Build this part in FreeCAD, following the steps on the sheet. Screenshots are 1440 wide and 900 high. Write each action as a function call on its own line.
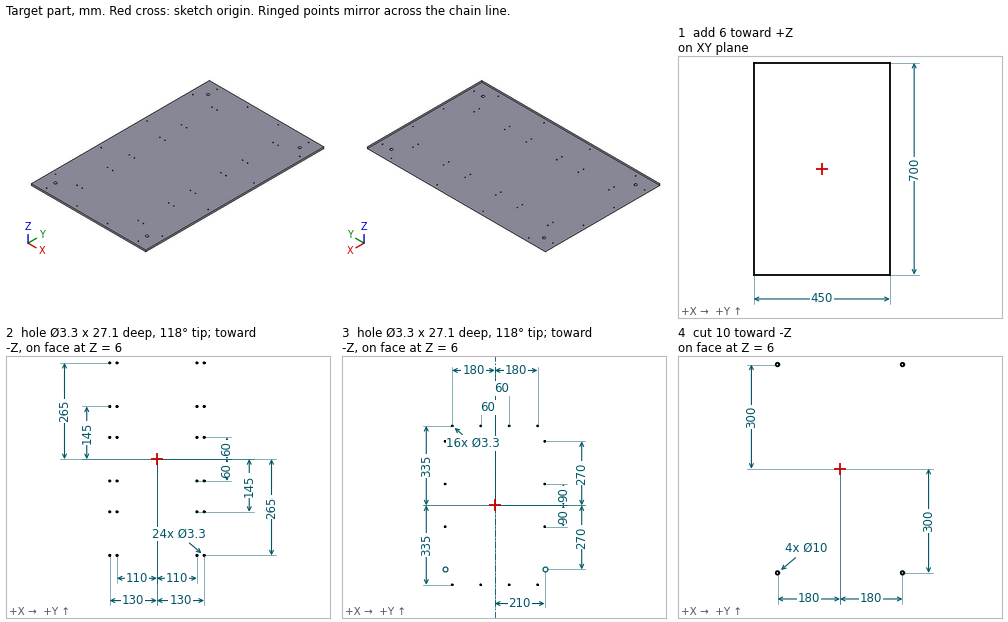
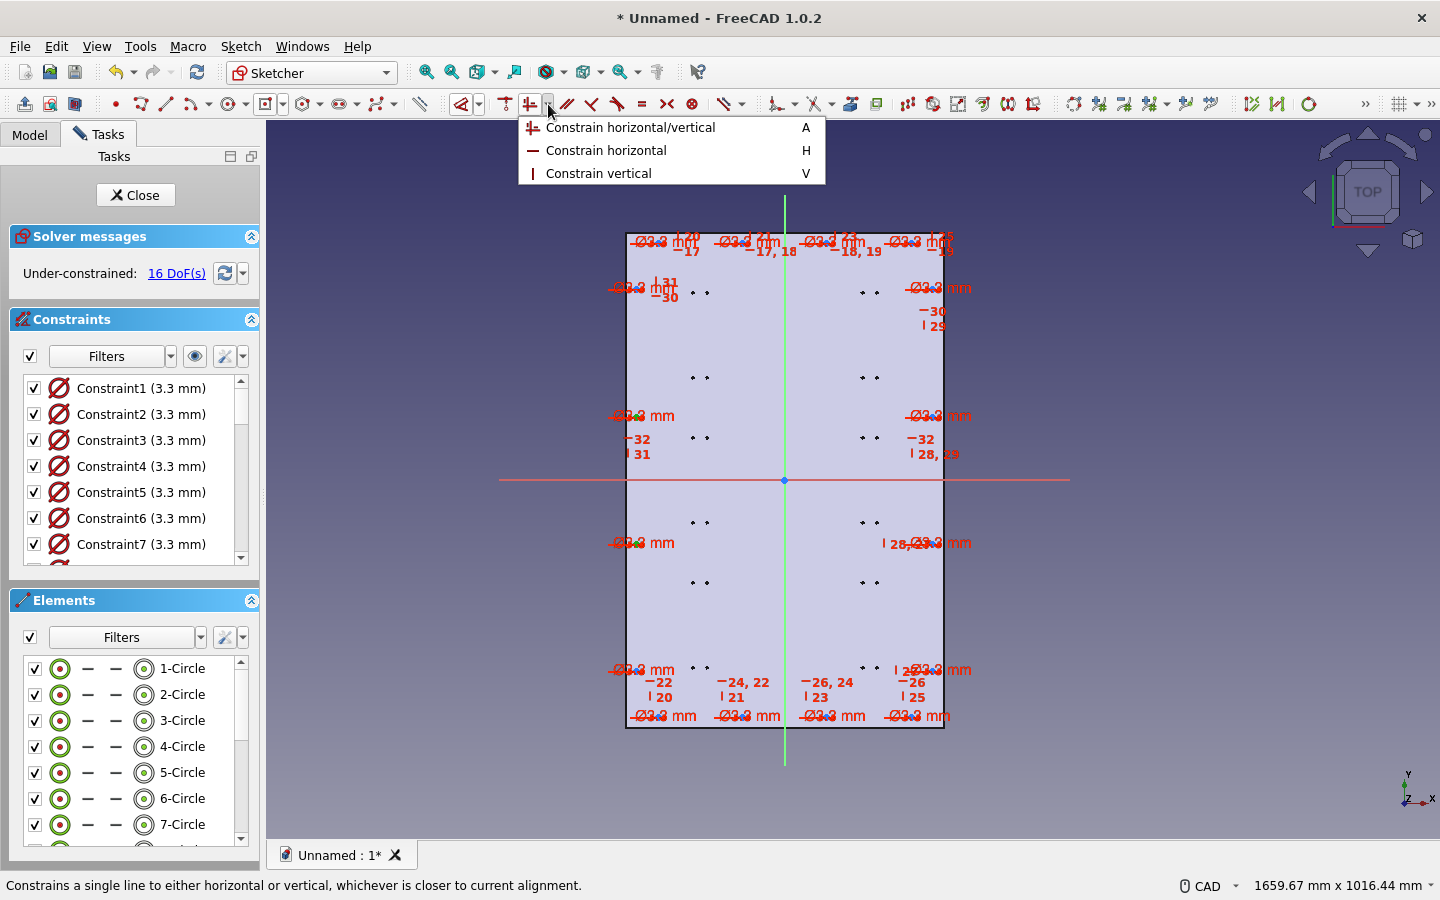
click(672, 174)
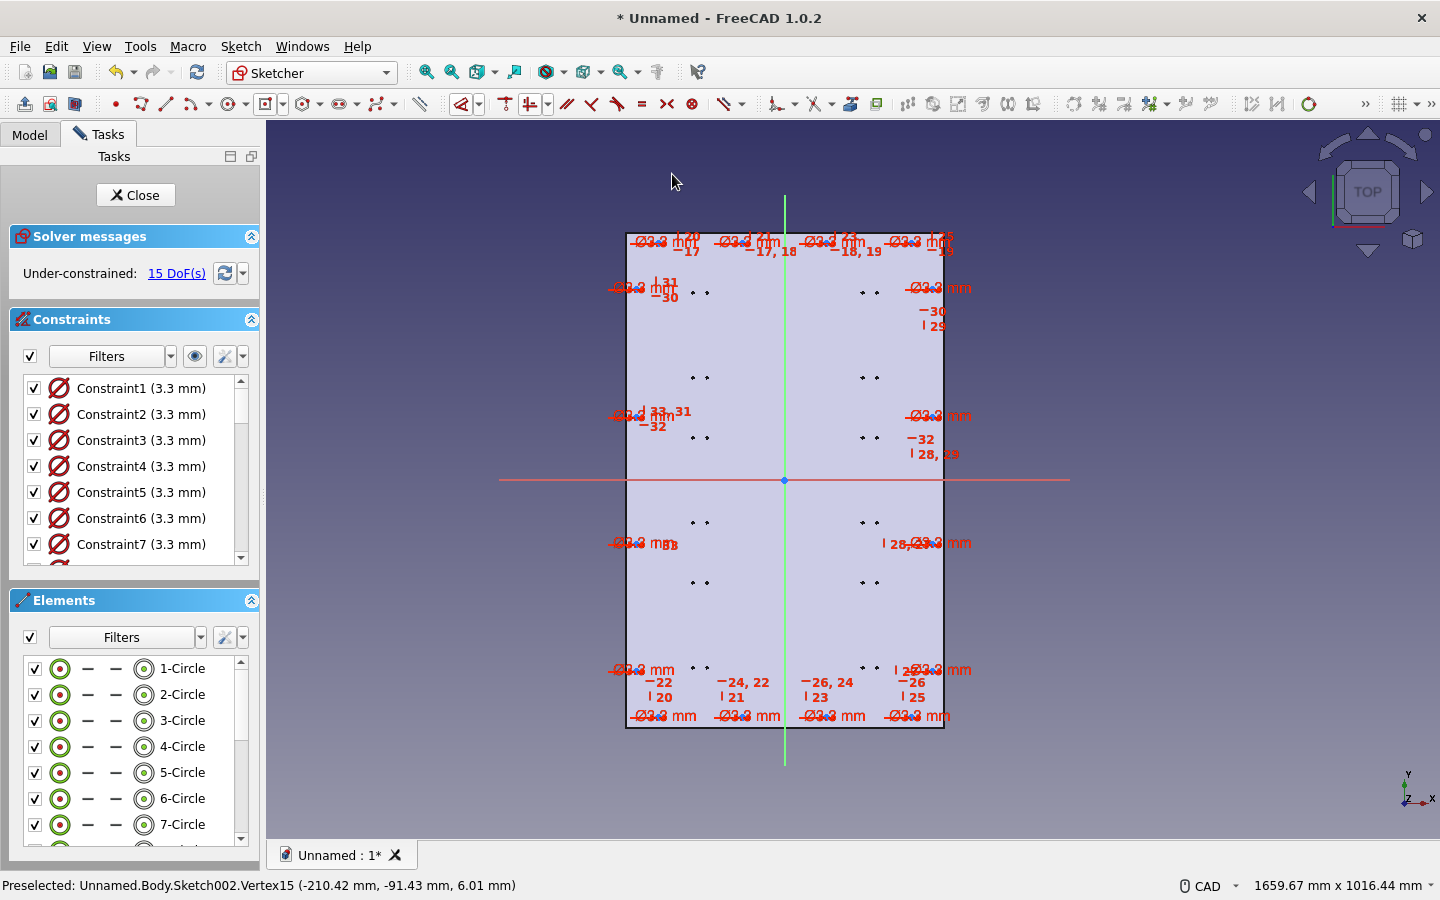
click(933, 545)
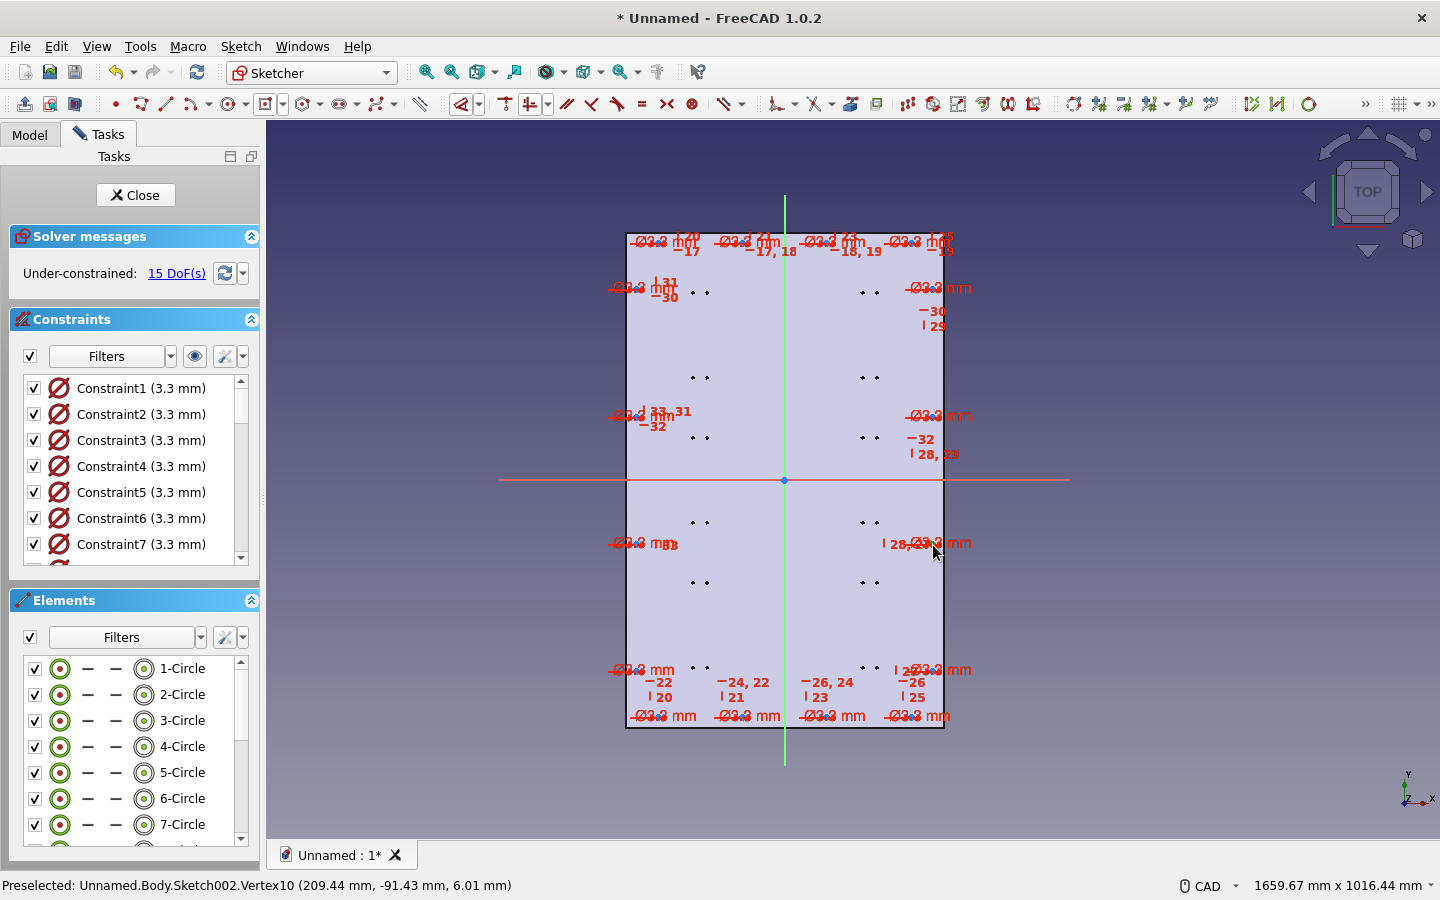
click(636, 545)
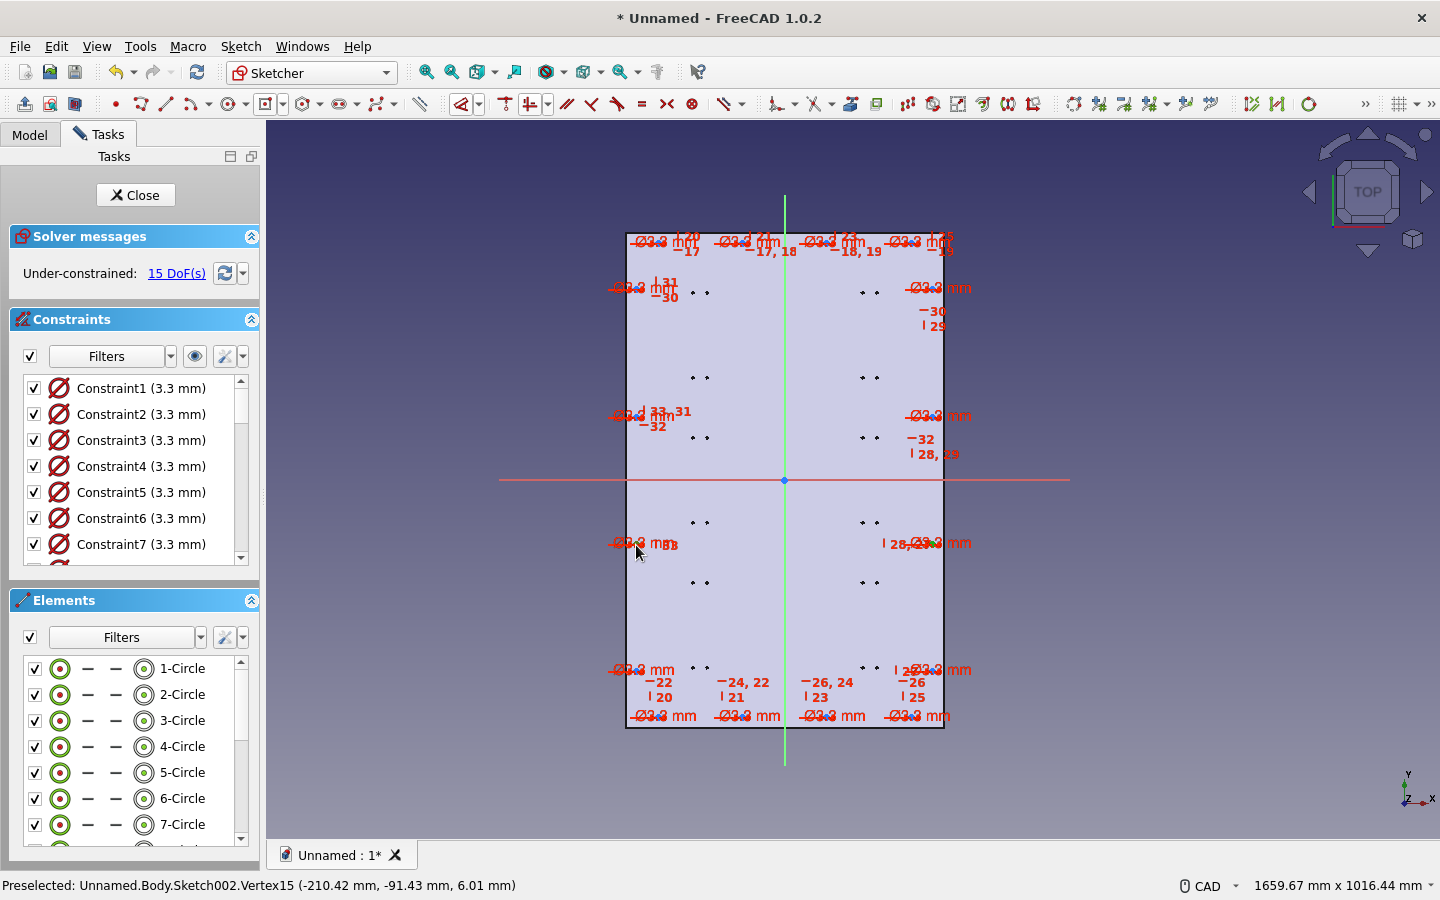
click(548, 104)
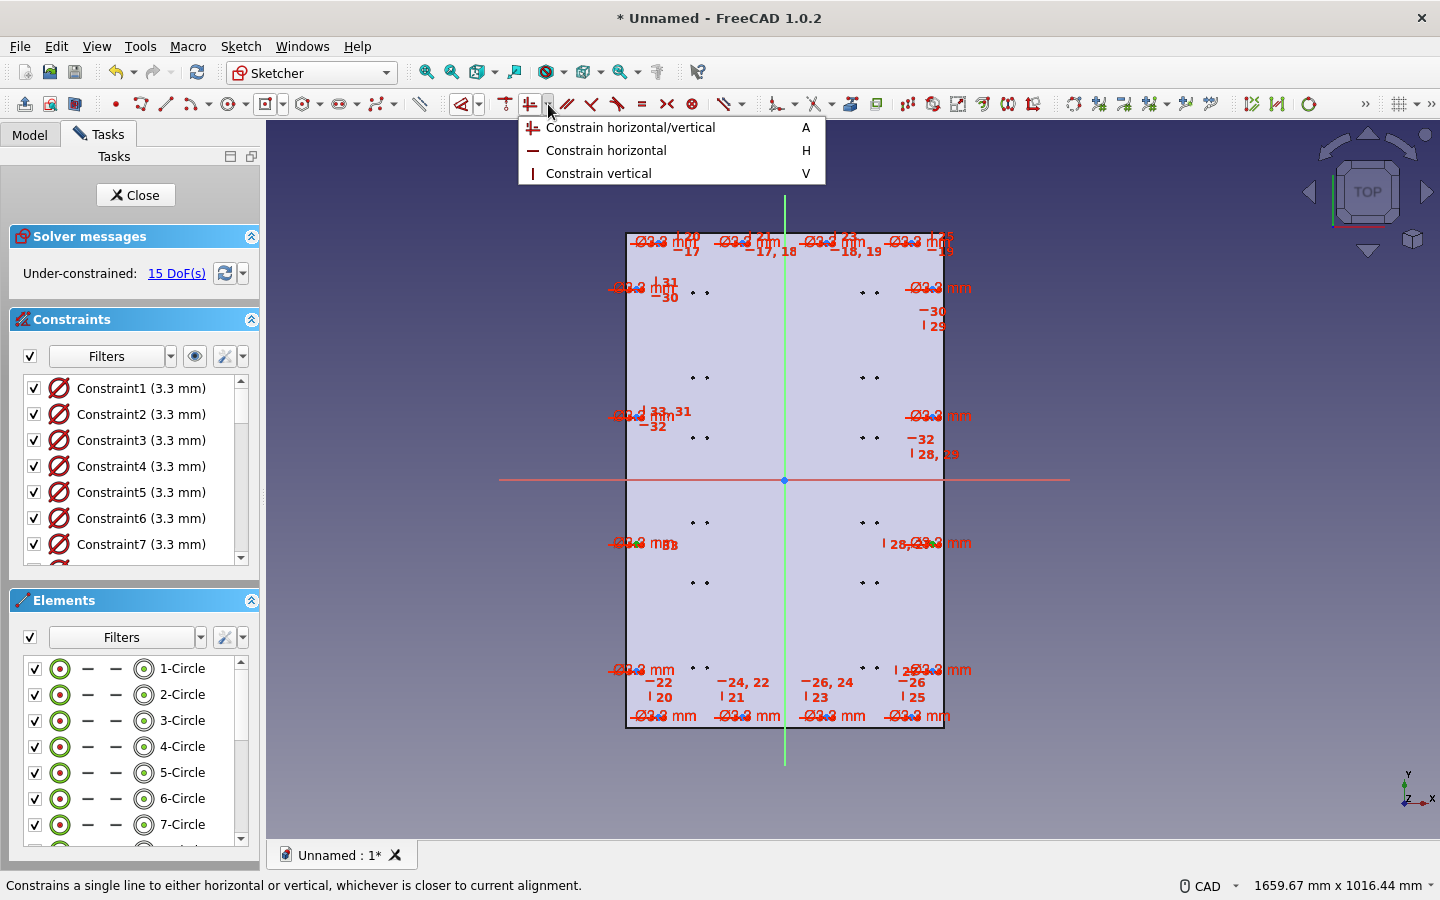
click(672, 150)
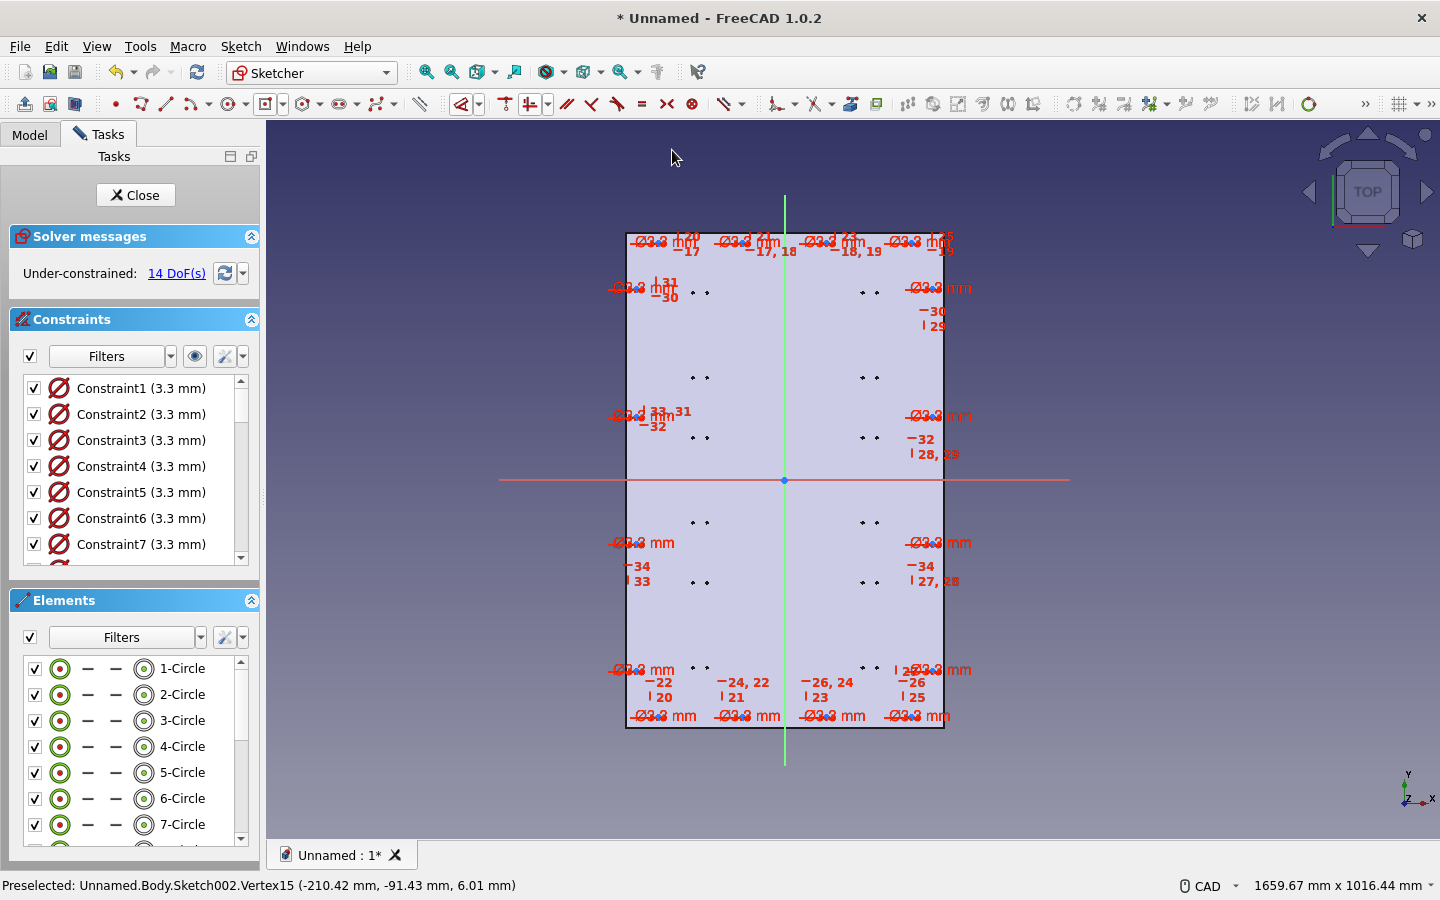
click(636, 545)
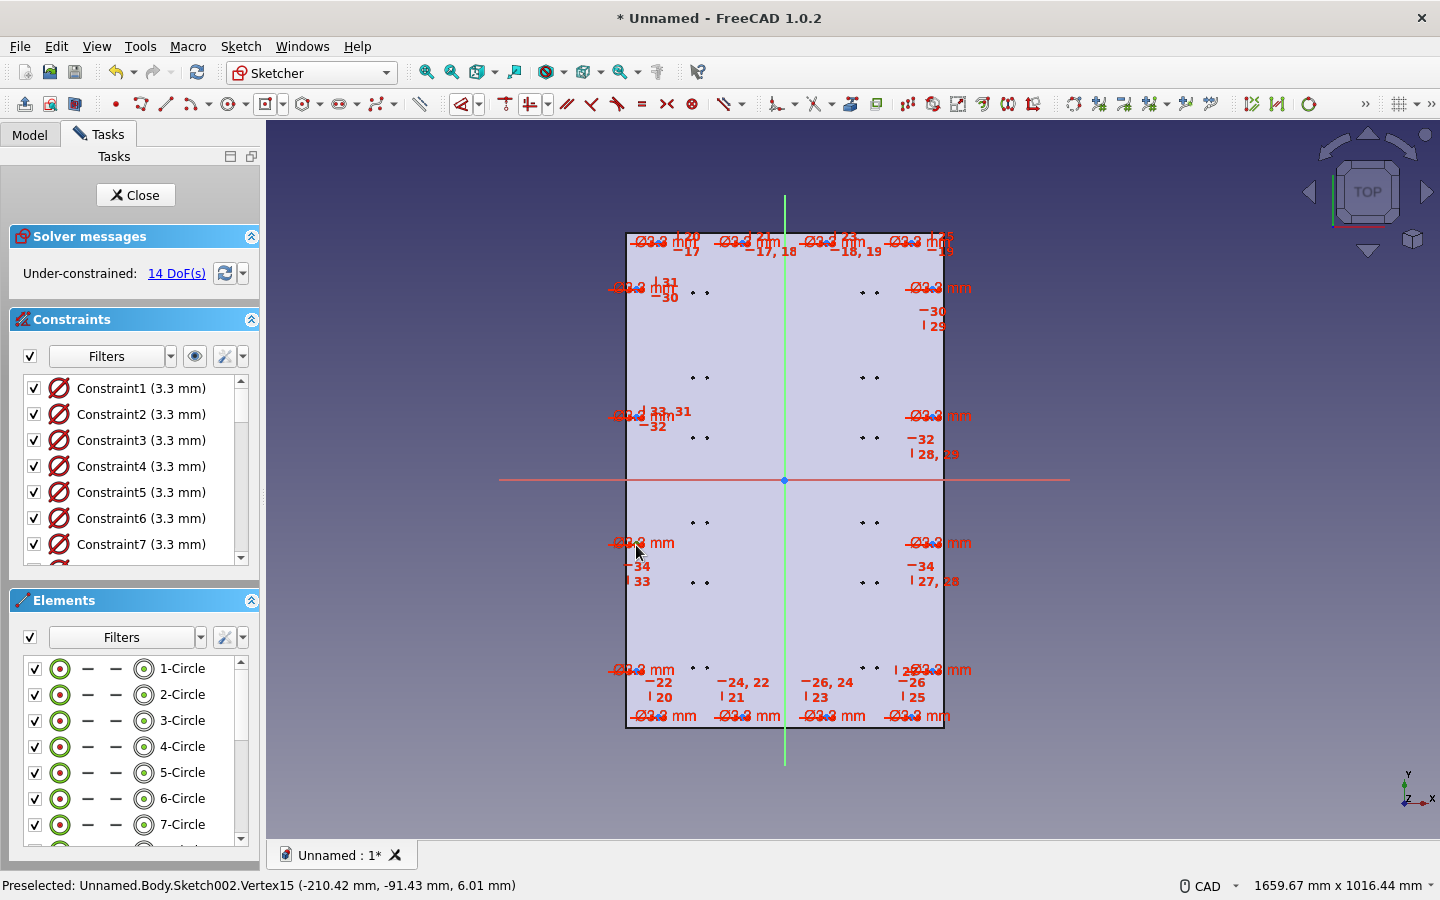
click(636, 672)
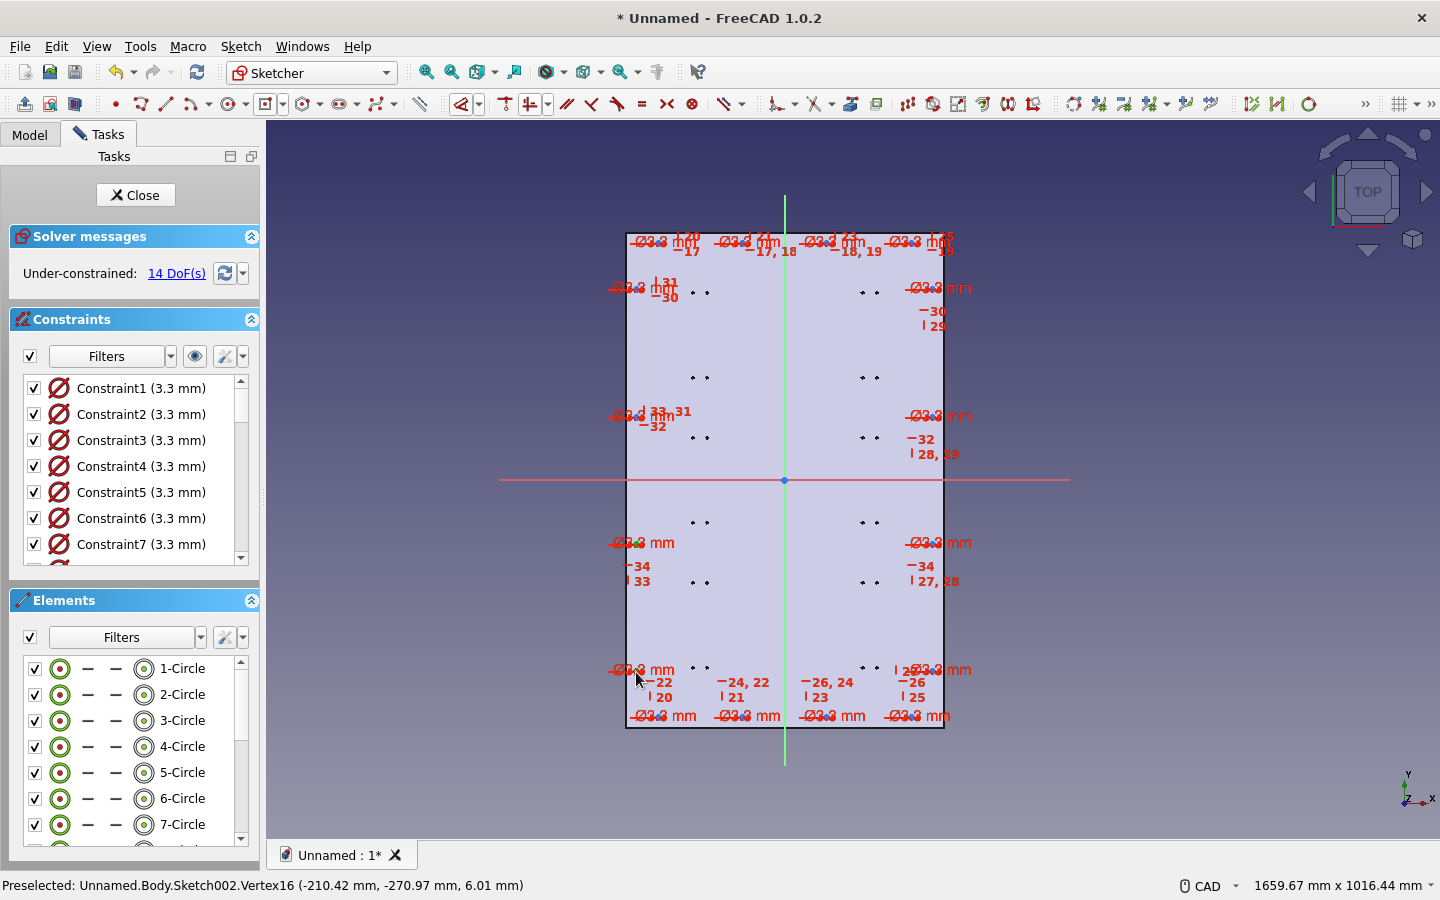
click(548, 104)